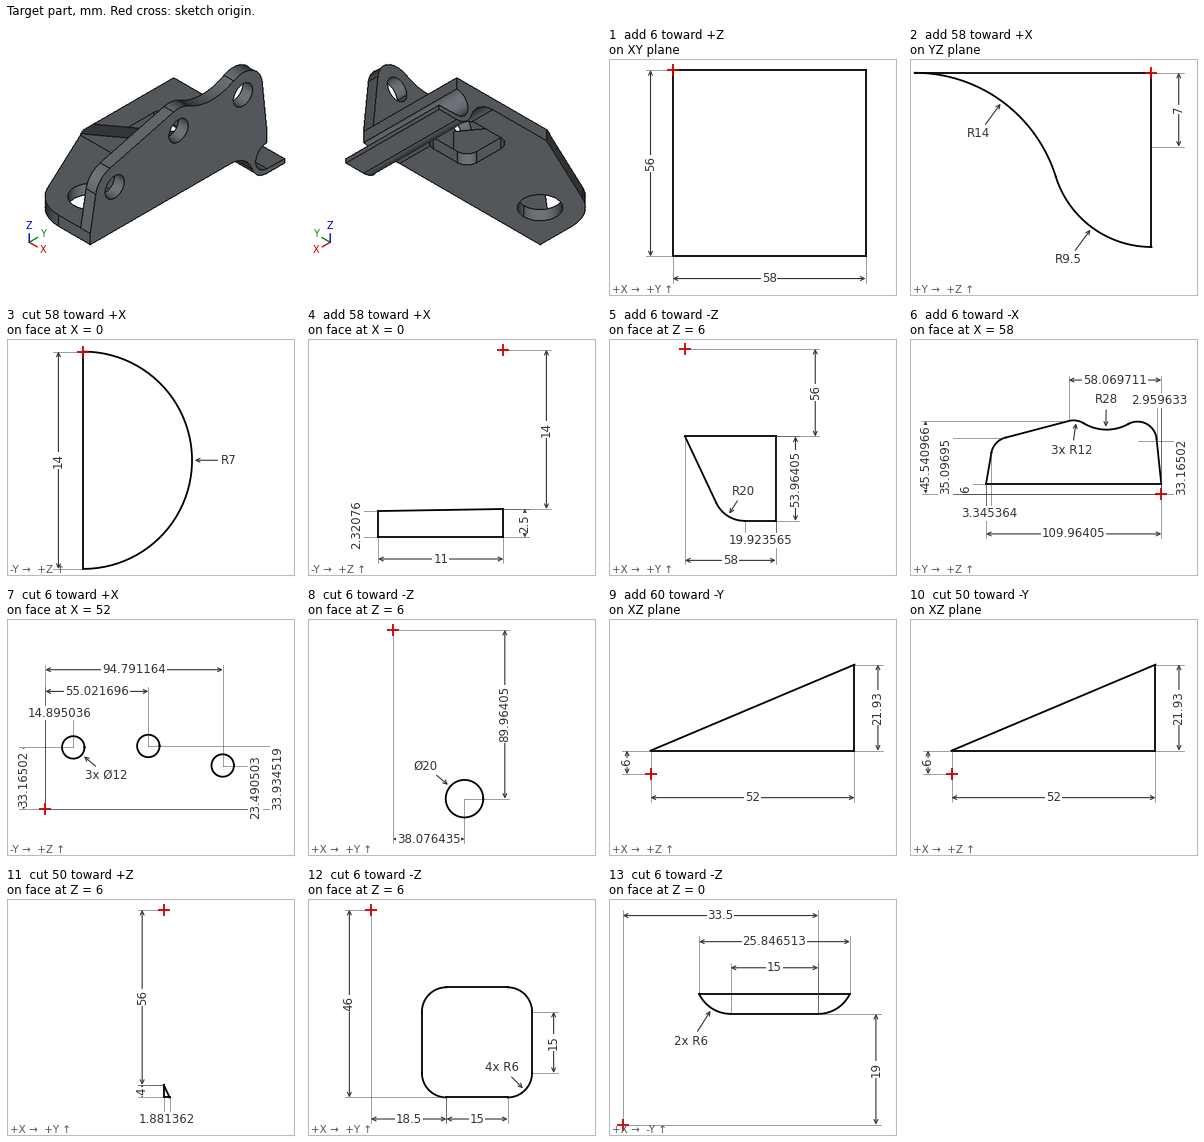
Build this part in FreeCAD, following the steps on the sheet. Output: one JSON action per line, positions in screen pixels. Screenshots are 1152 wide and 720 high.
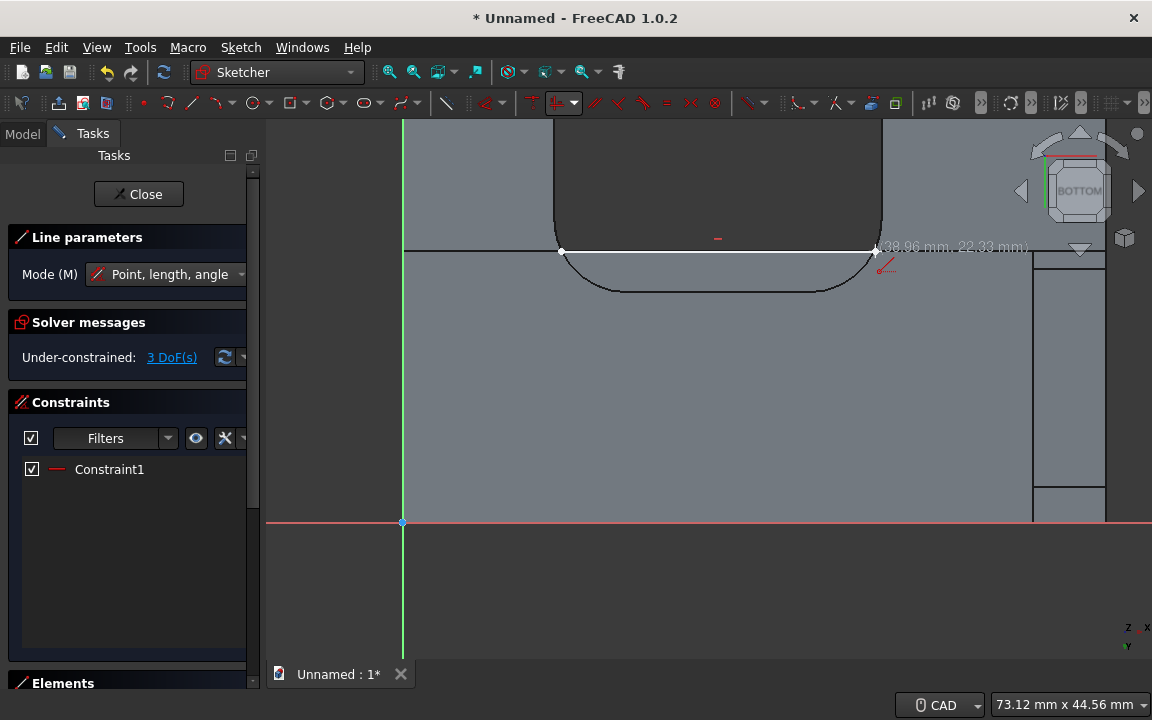
{"action": "left_click", "coordinate": [809, 292]}
{"action": "left_click", "coordinate": [627, 292]}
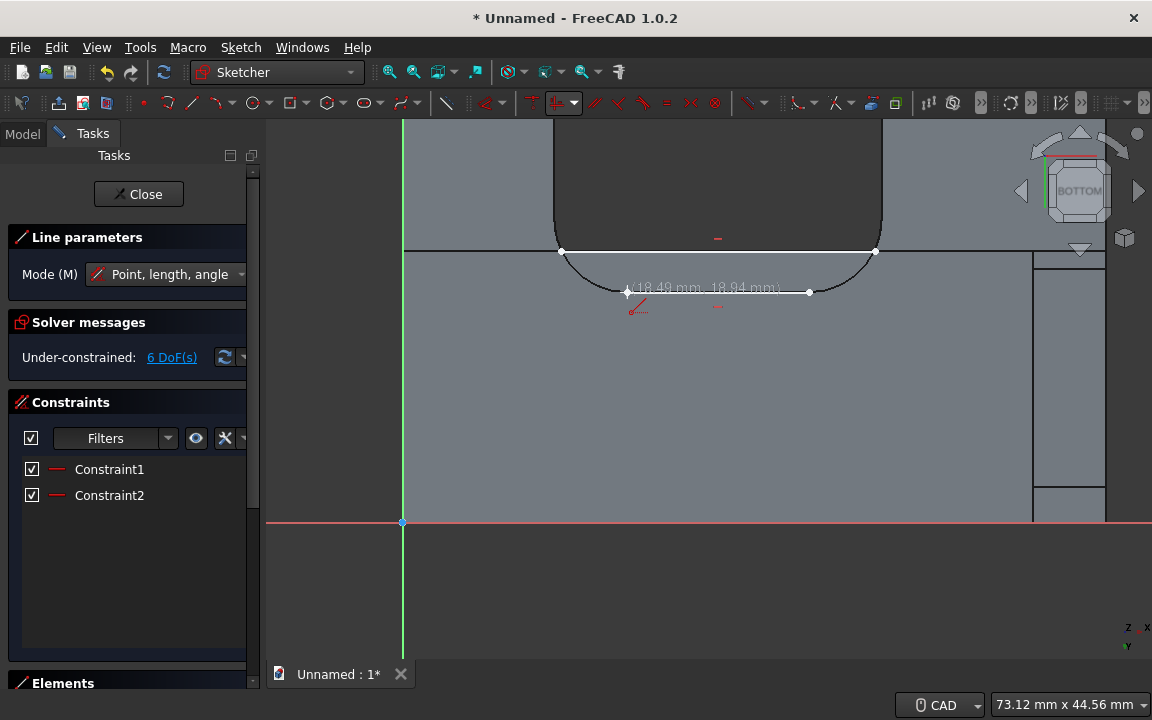
{"action": "left_click", "coordinate": [216, 104]}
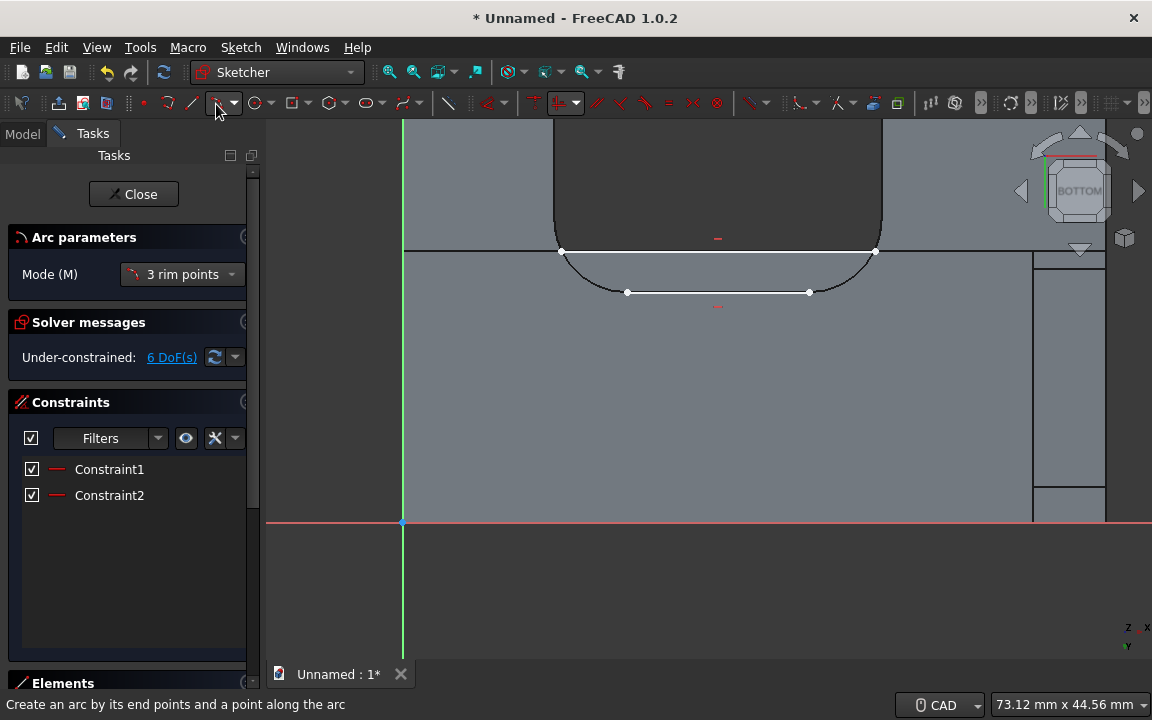
{"action": "left_click", "coordinate": [875, 252]}
{"action": "left_click", "coordinate": [809, 293]}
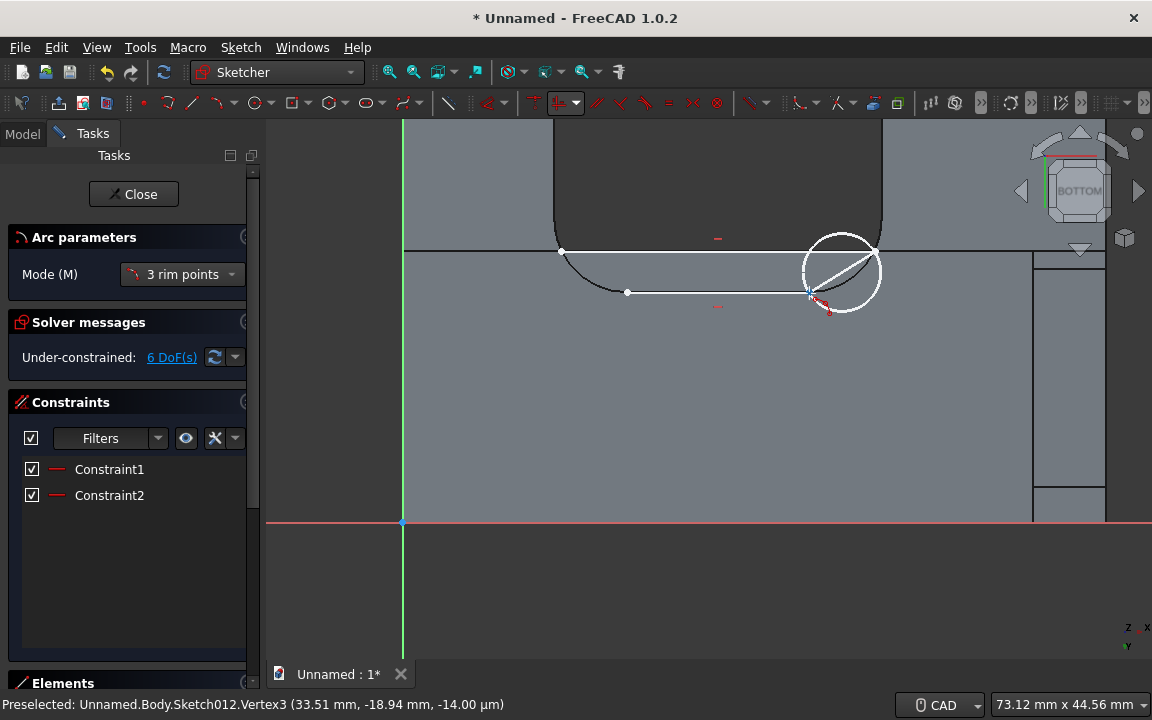
{"action": "scroll", "coordinate": [848, 281], "scroll_direction": "up", "scroll_amount": 2}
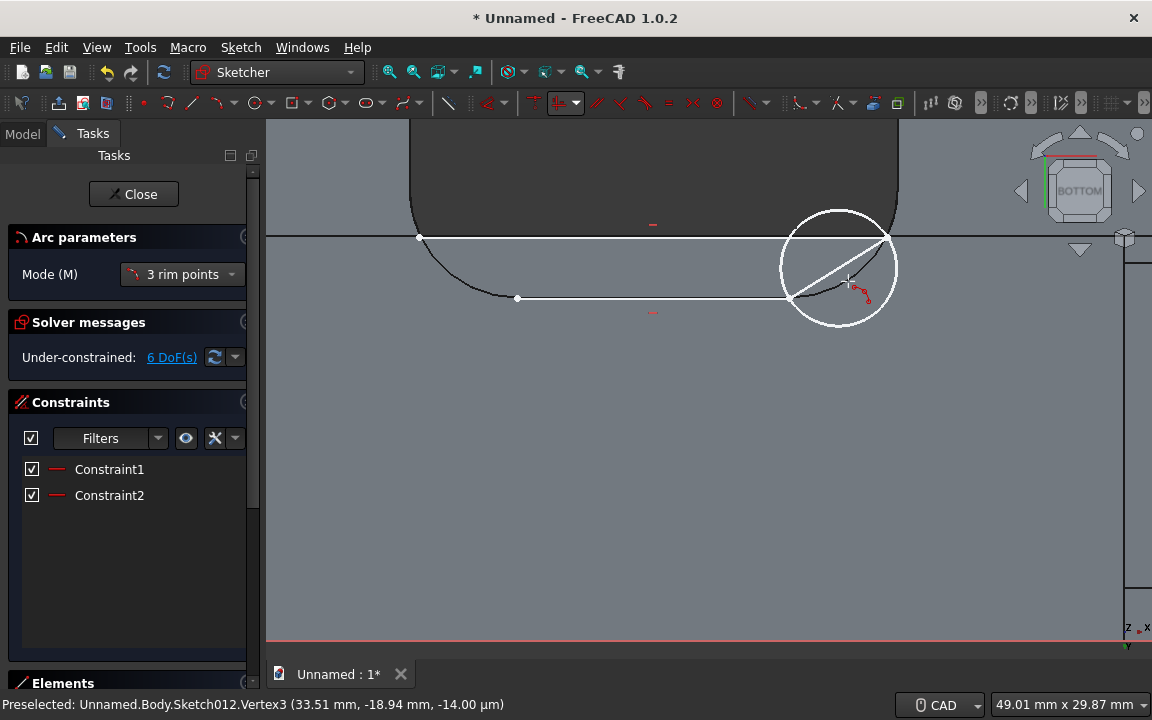
{"action": "left_click", "coordinate": [847, 281]}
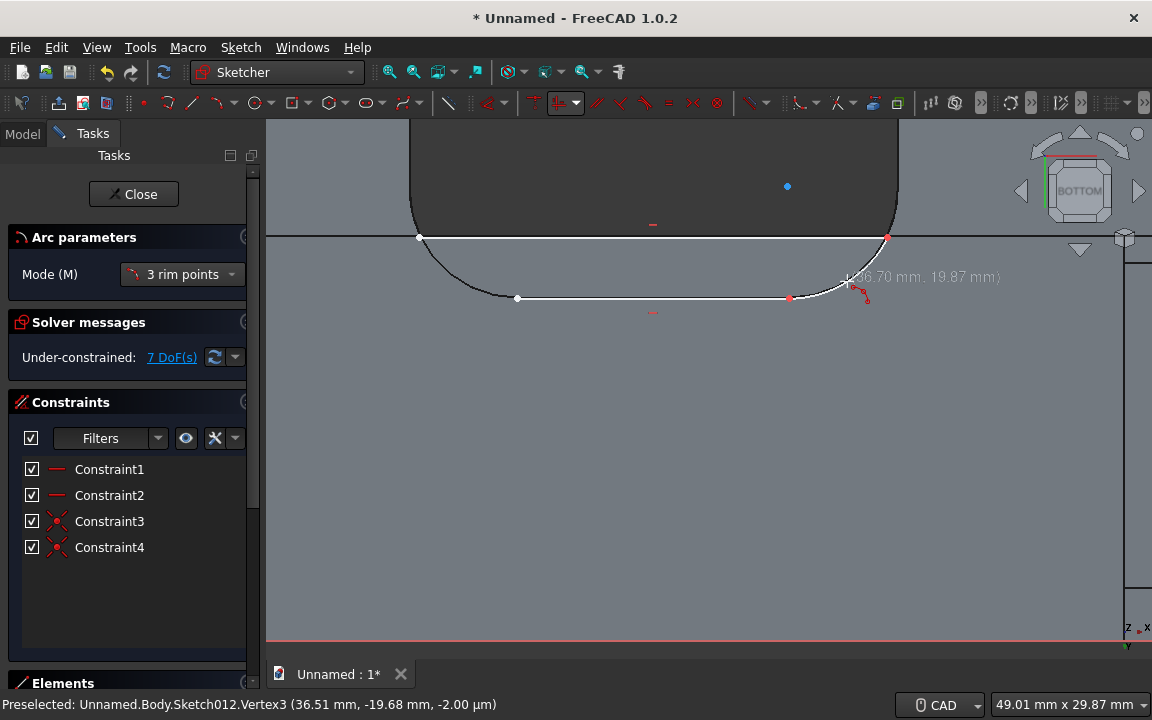
{"action": "left_click", "coordinate": [518, 299]}
{"action": "left_click", "coordinate": [420, 238]}
{"action": "left_click", "coordinate": [460, 281]}
{"action": "key", "text": "Escape"}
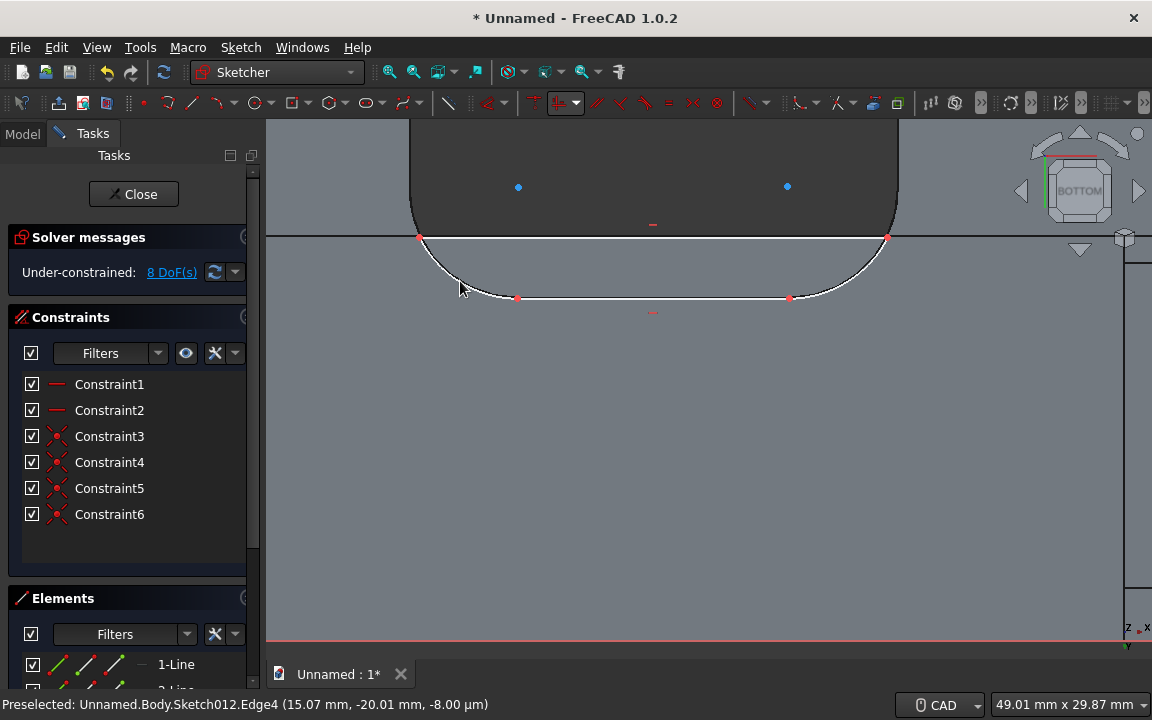
{"action": "left_click", "coordinate": [708, 299]}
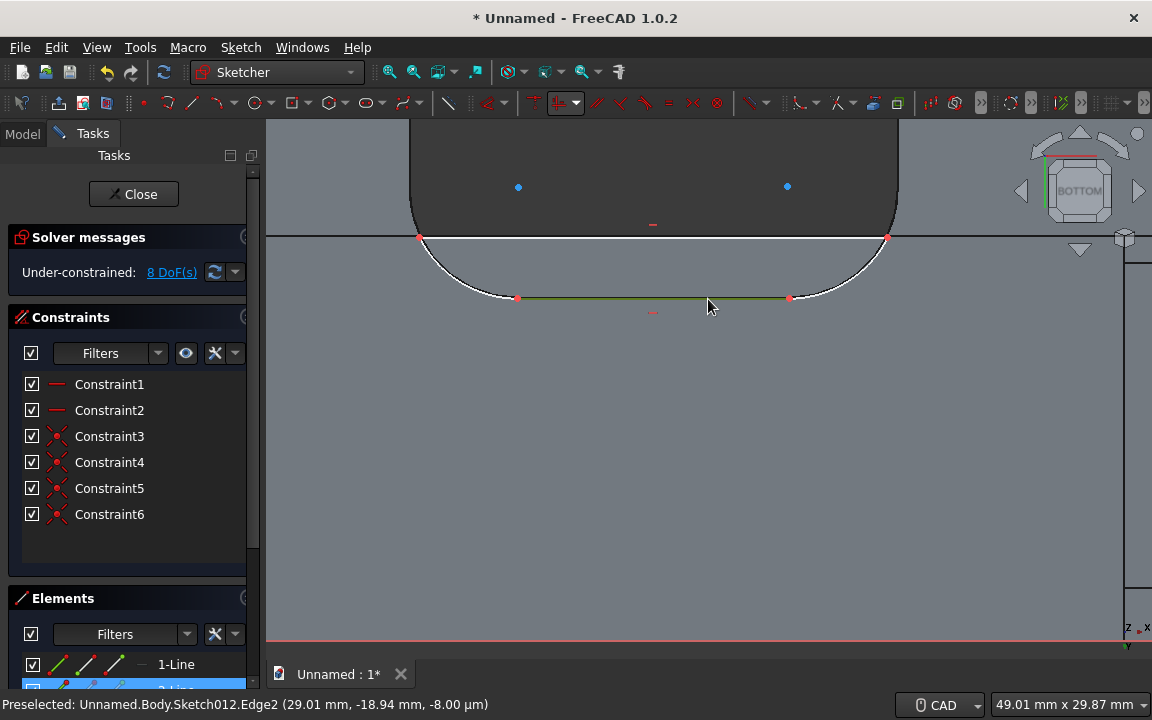
{"action": "left_click", "coordinate": [825, 292]}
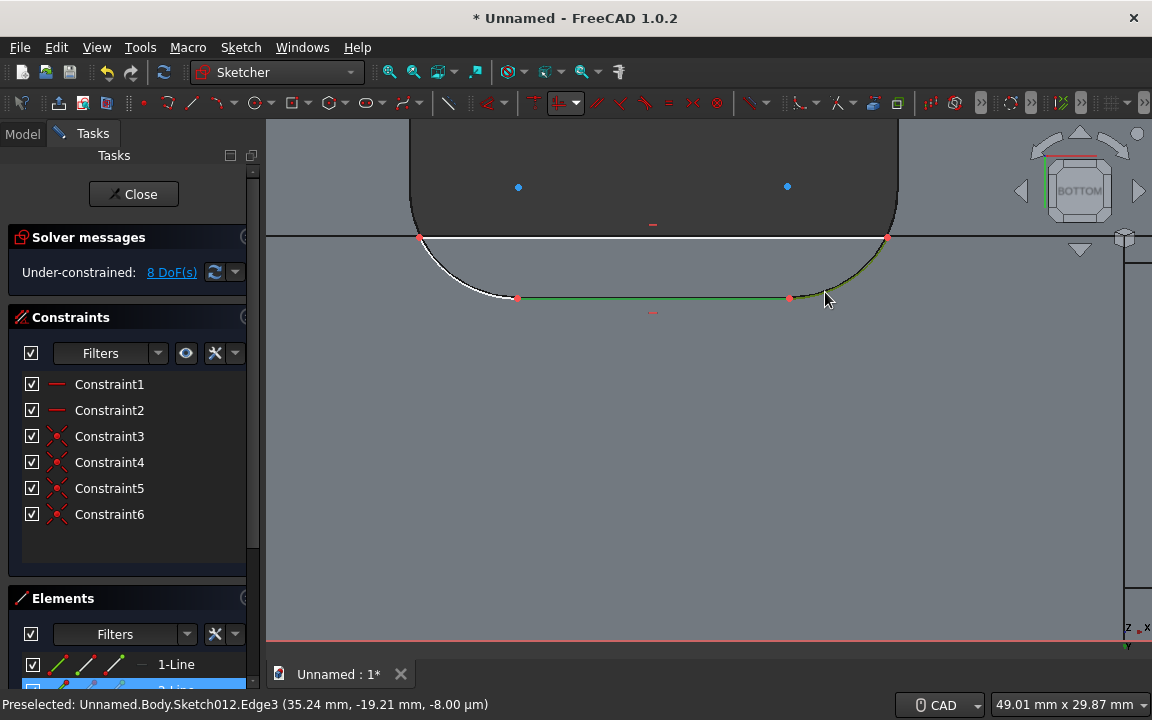
{"action": "left_click", "coordinate": [646, 104]}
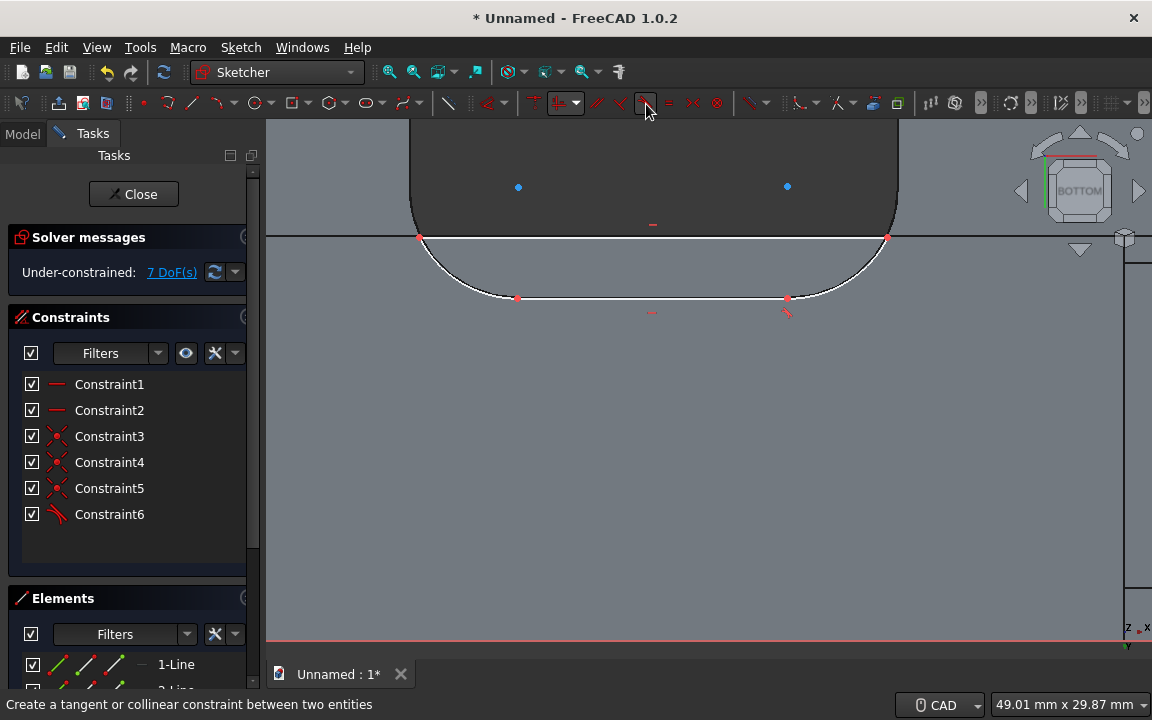
{"action": "left_click", "coordinate": [707, 299]}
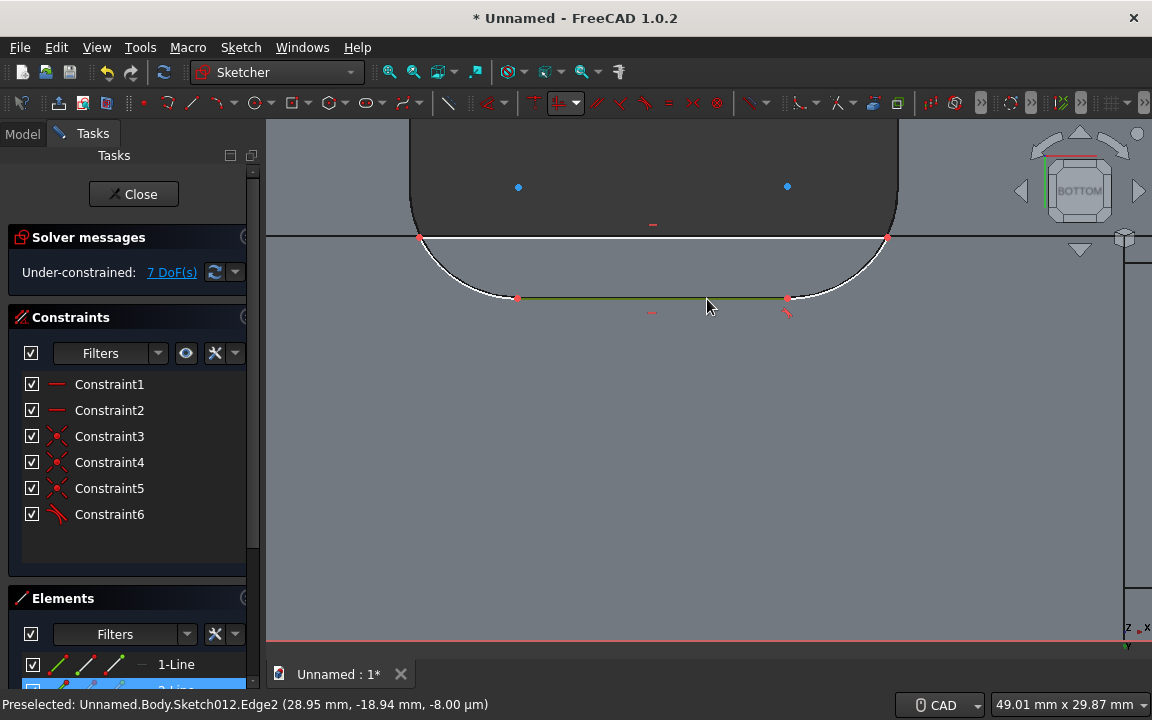
{"action": "left_click", "coordinate": [441, 267]}